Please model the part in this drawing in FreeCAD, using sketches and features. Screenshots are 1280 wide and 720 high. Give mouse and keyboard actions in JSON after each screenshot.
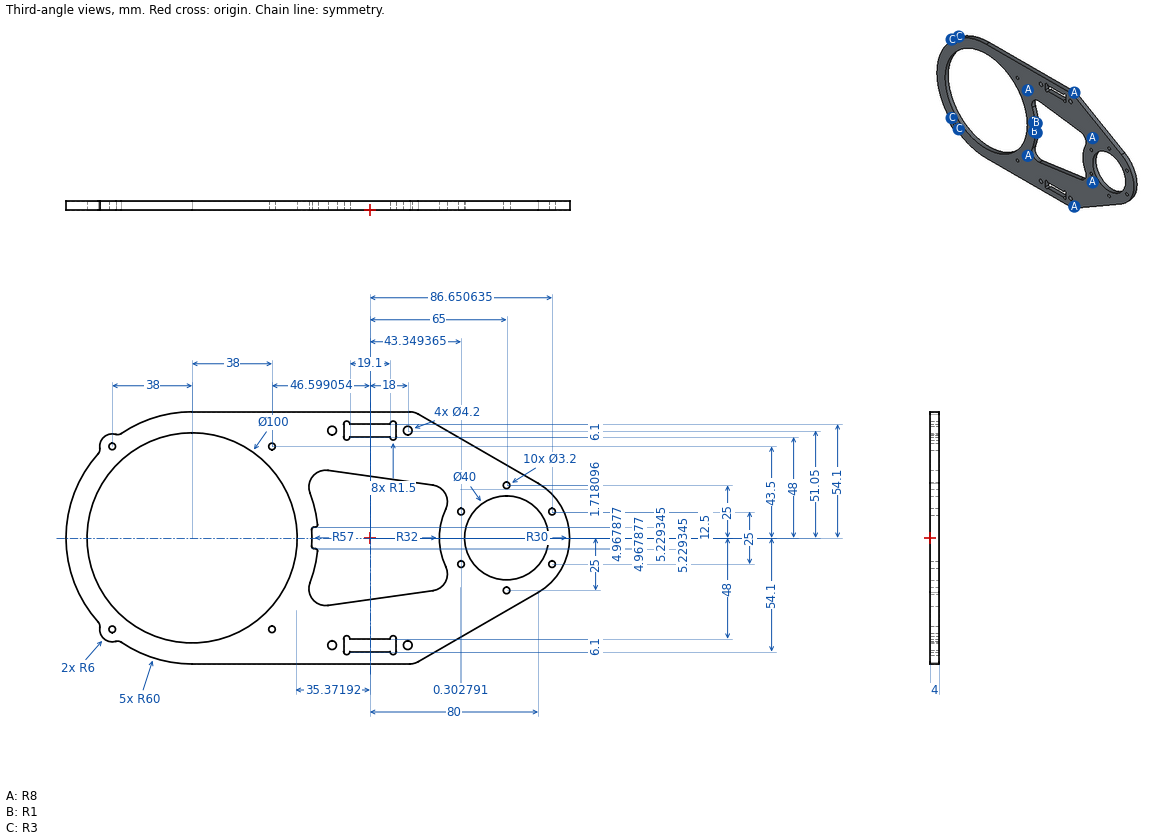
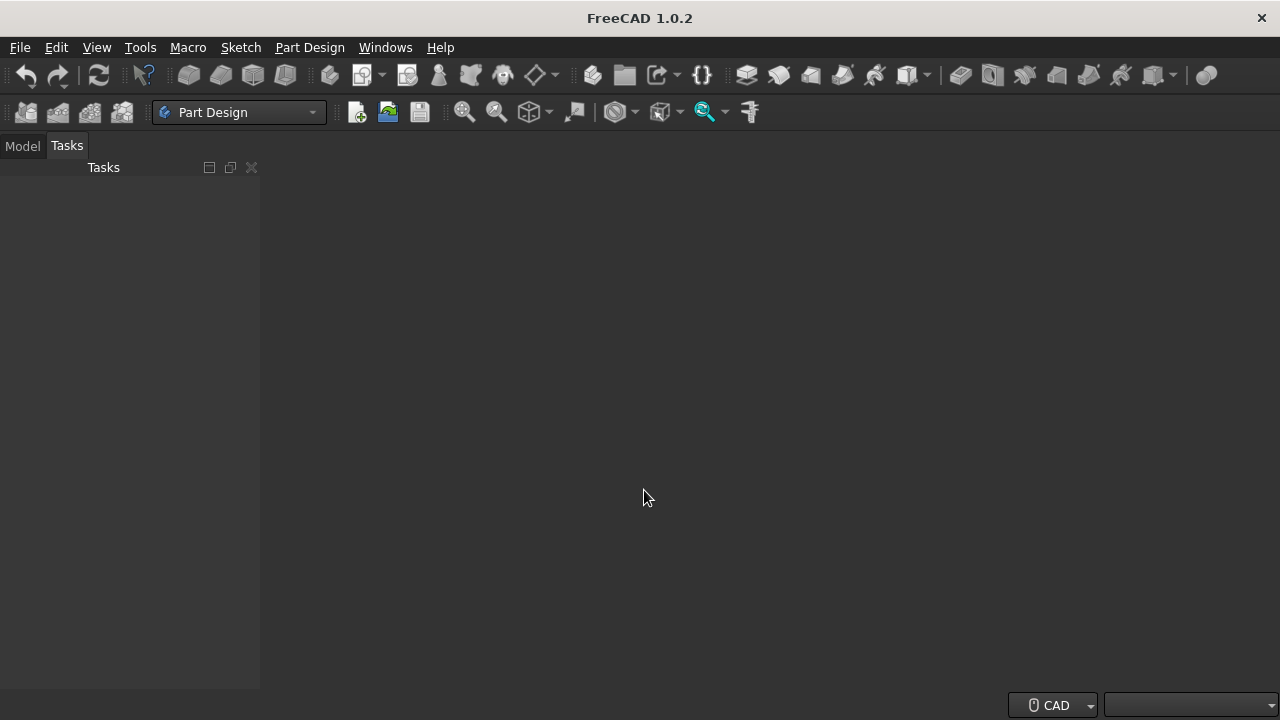
{"action": "left_click", "coordinate": [356, 112]}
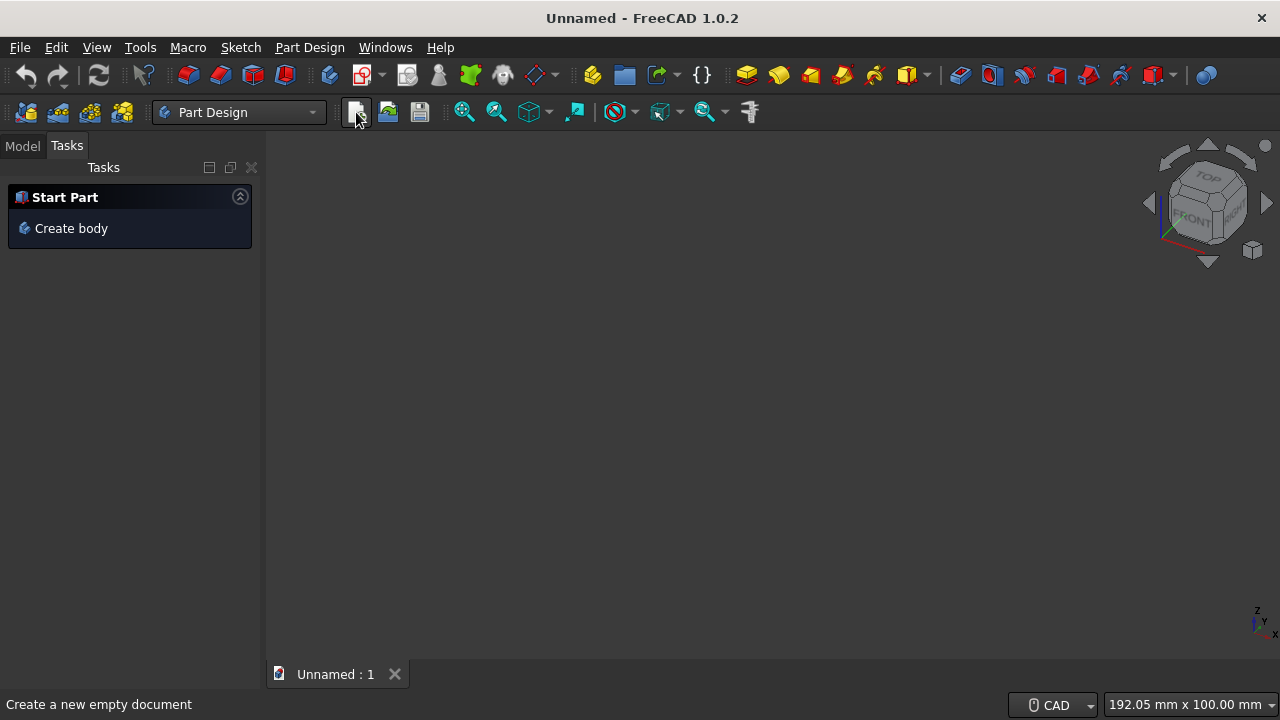
{"action": "left_click", "coordinate": [362, 76]}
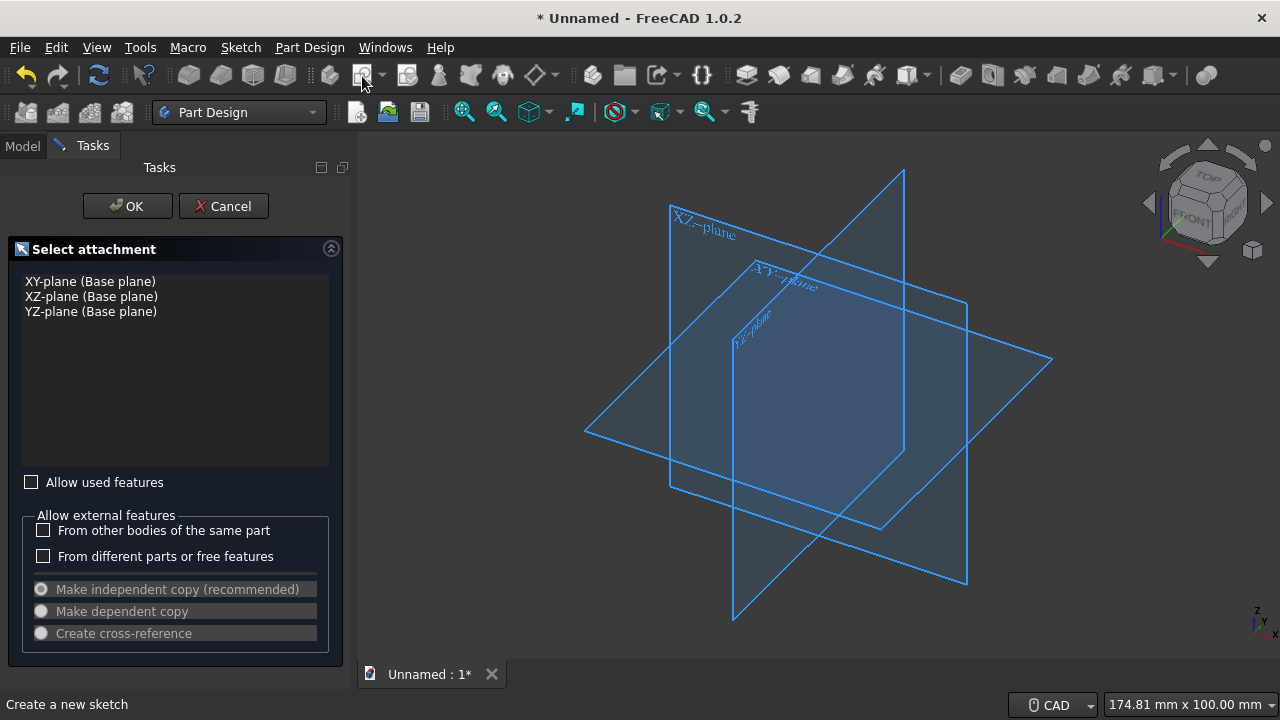
{"action": "left_click", "coordinate": [82, 296]}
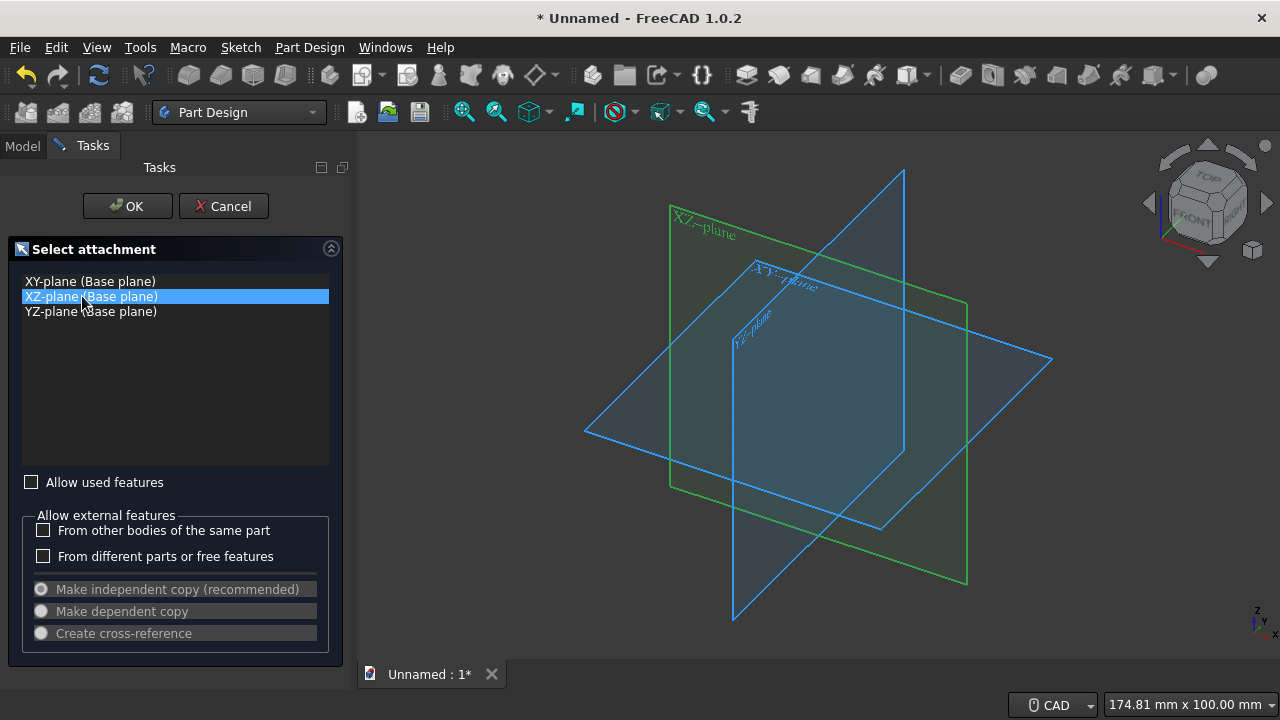
{"action": "left_click", "coordinate": [128, 206]}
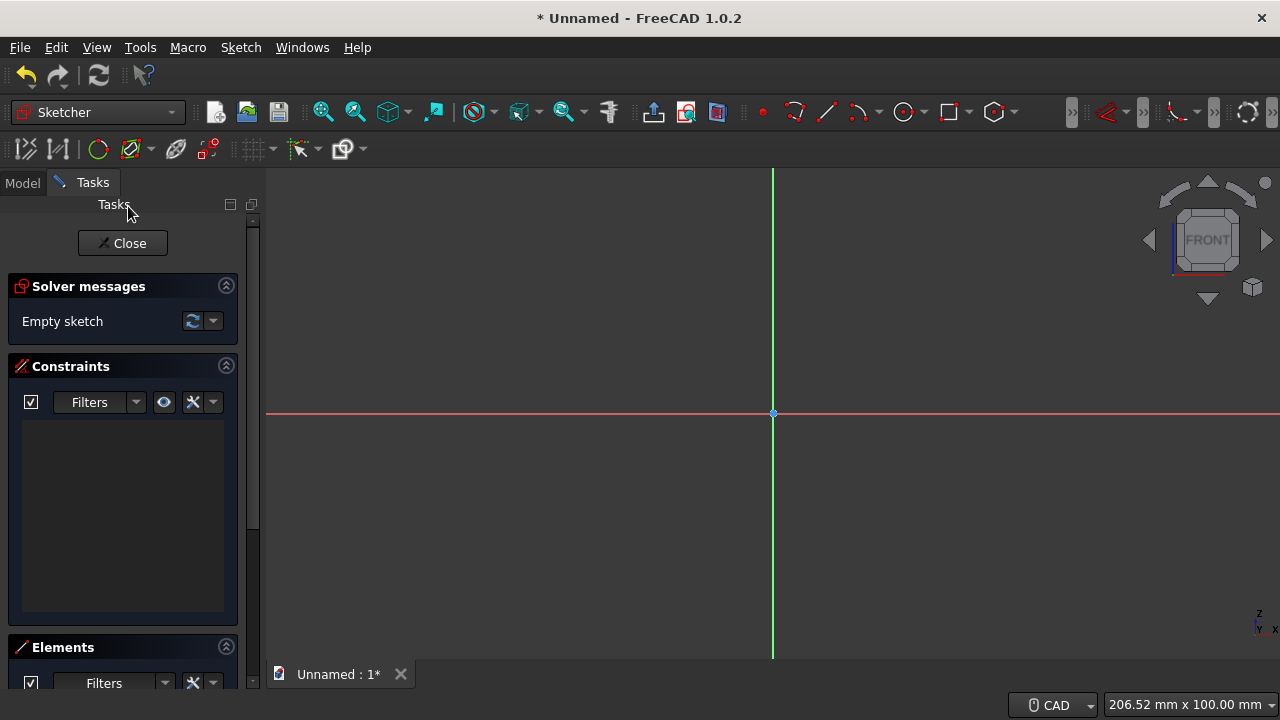
{"action": "scroll", "coordinate": [748, 414], "scroll_direction": "down", "scroll_amount": 4}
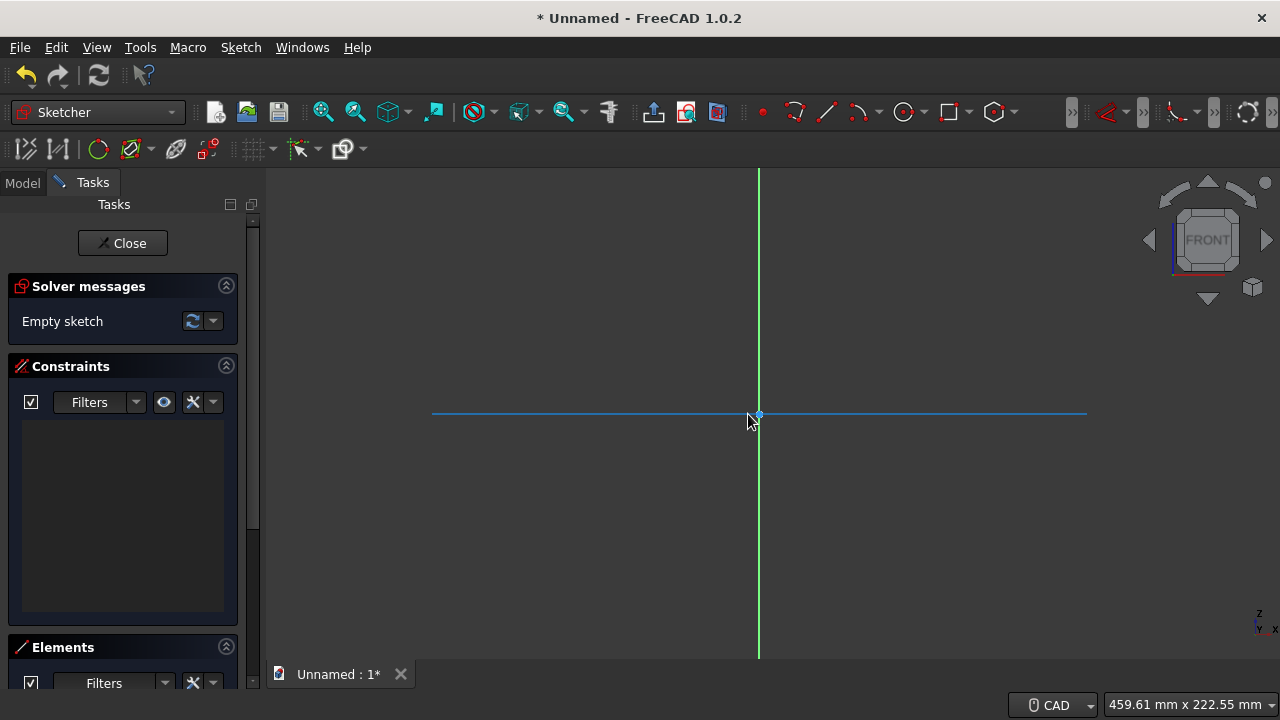
{"action": "left_click", "coordinate": [796, 112]}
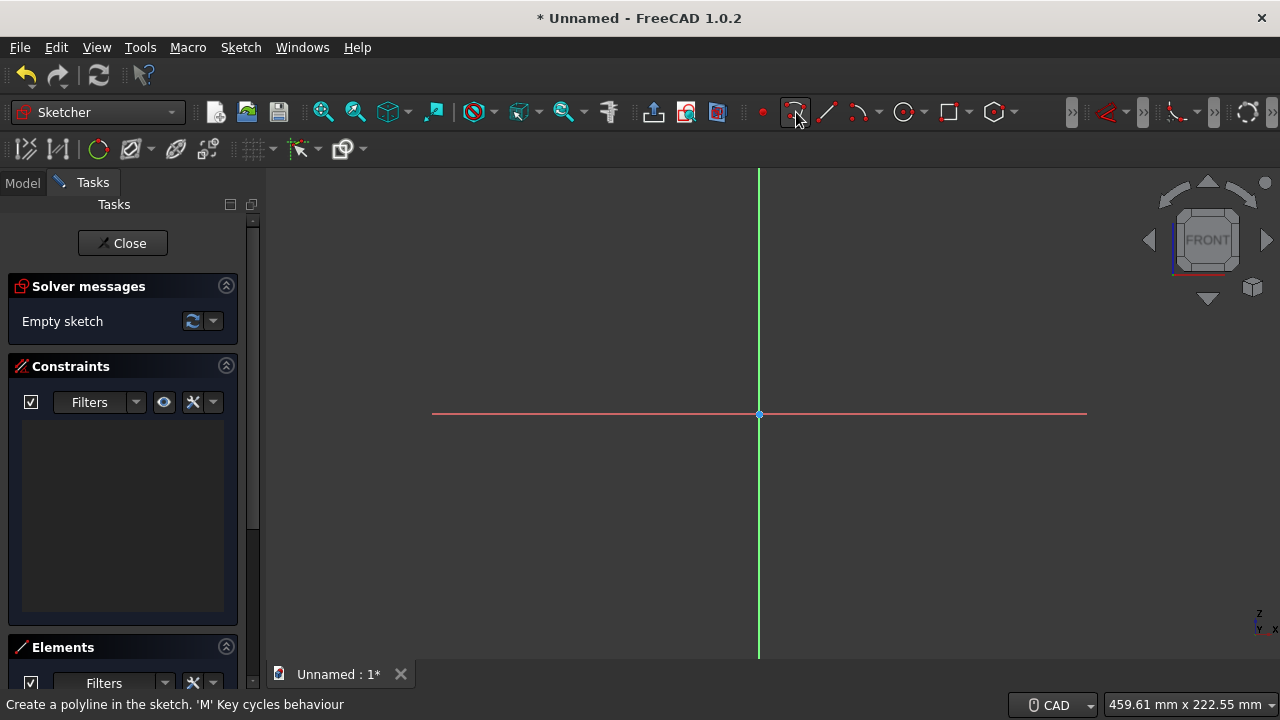
{"action": "left_click", "coordinate": [936, 471]}
{"action": "left_click", "coordinate": [806, 546]}
{"action": "left_click", "coordinate": [573, 546]}
{"action": "right_click", "coordinate": [573, 546]}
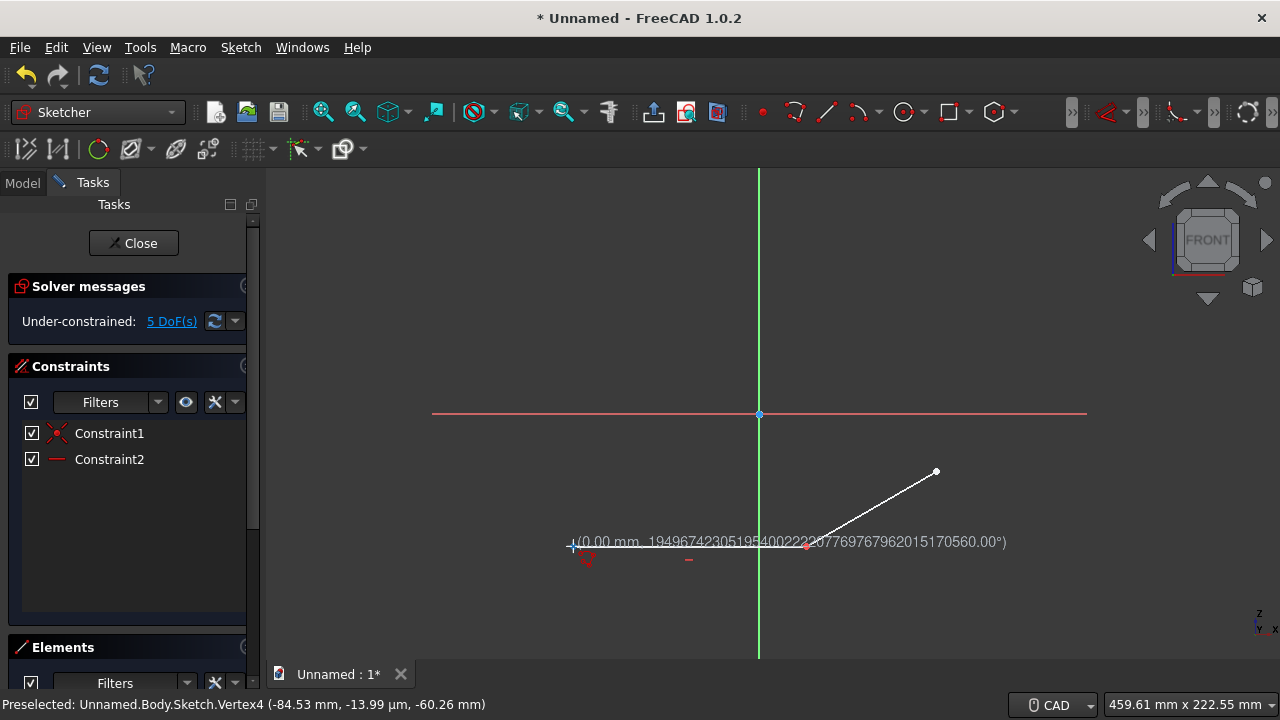
{"action": "left_click", "coordinate": [573, 282]}
{"action": "left_click", "coordinate": [806, 282]}
{"action": "left_click", "coordinate": [936, 357]}
{"action": "right_click", "coordinate": [936, 357]}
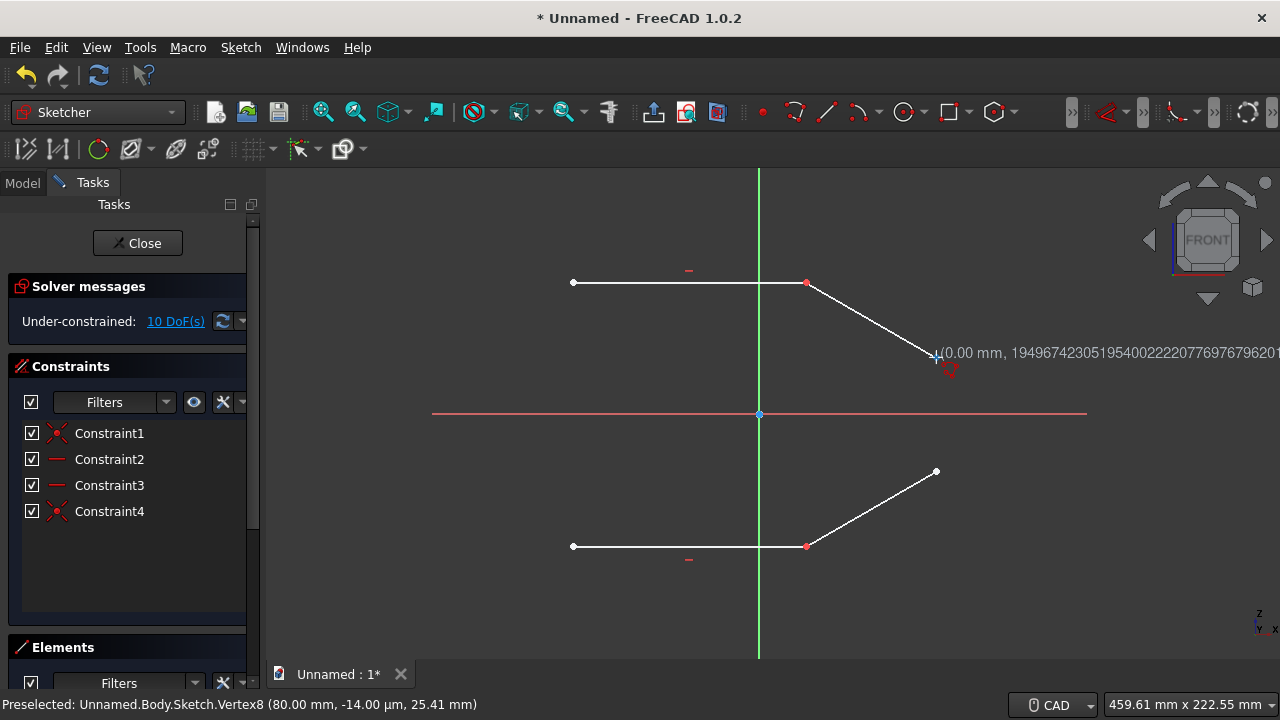
{"action": "left_click", "coordinate": [882, 112]}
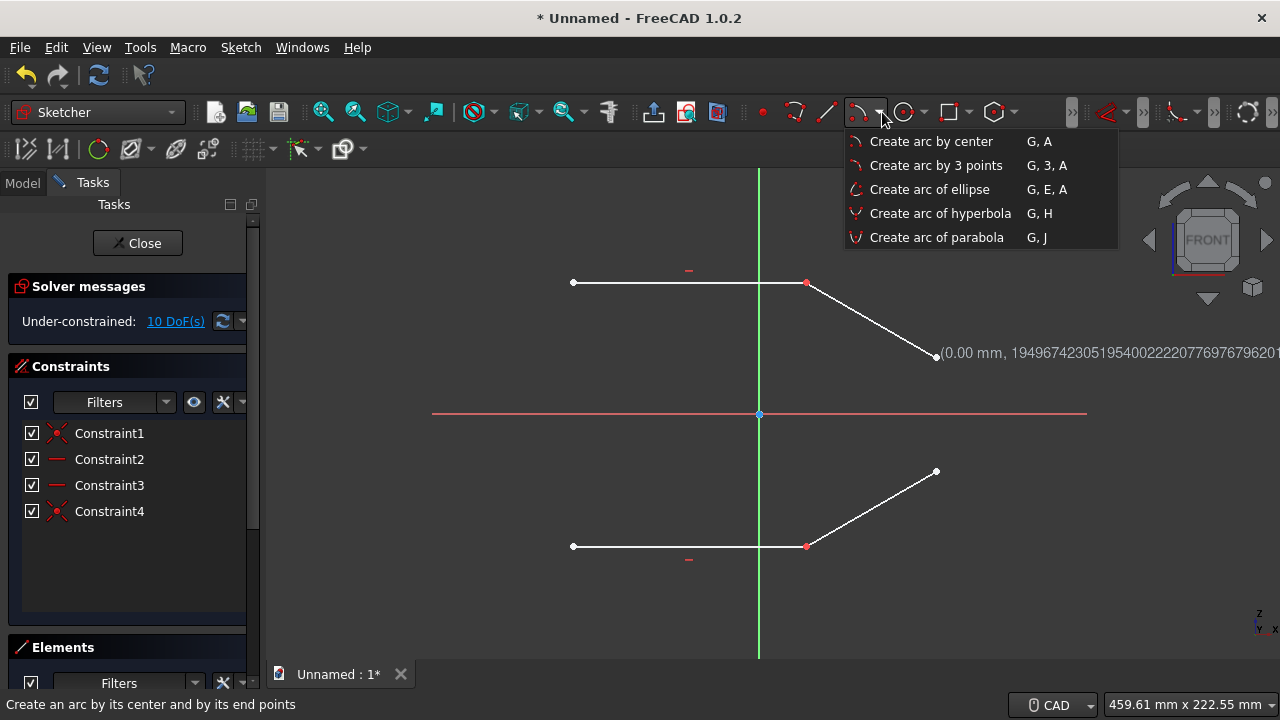
{"action": "left_click", "coordinate": [982, 165]}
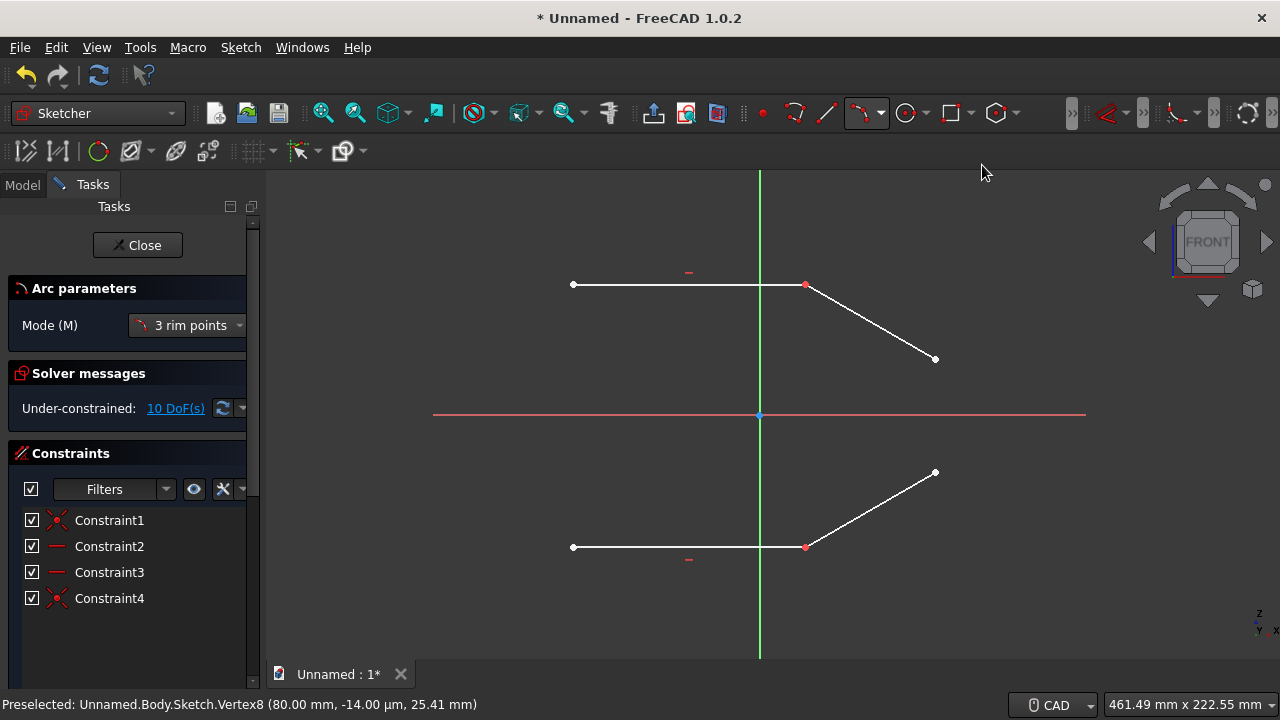
{"action": "left_click", "coordinate": [574, 547]}
{"action": "left_click", "coordinate": [497, 522]}